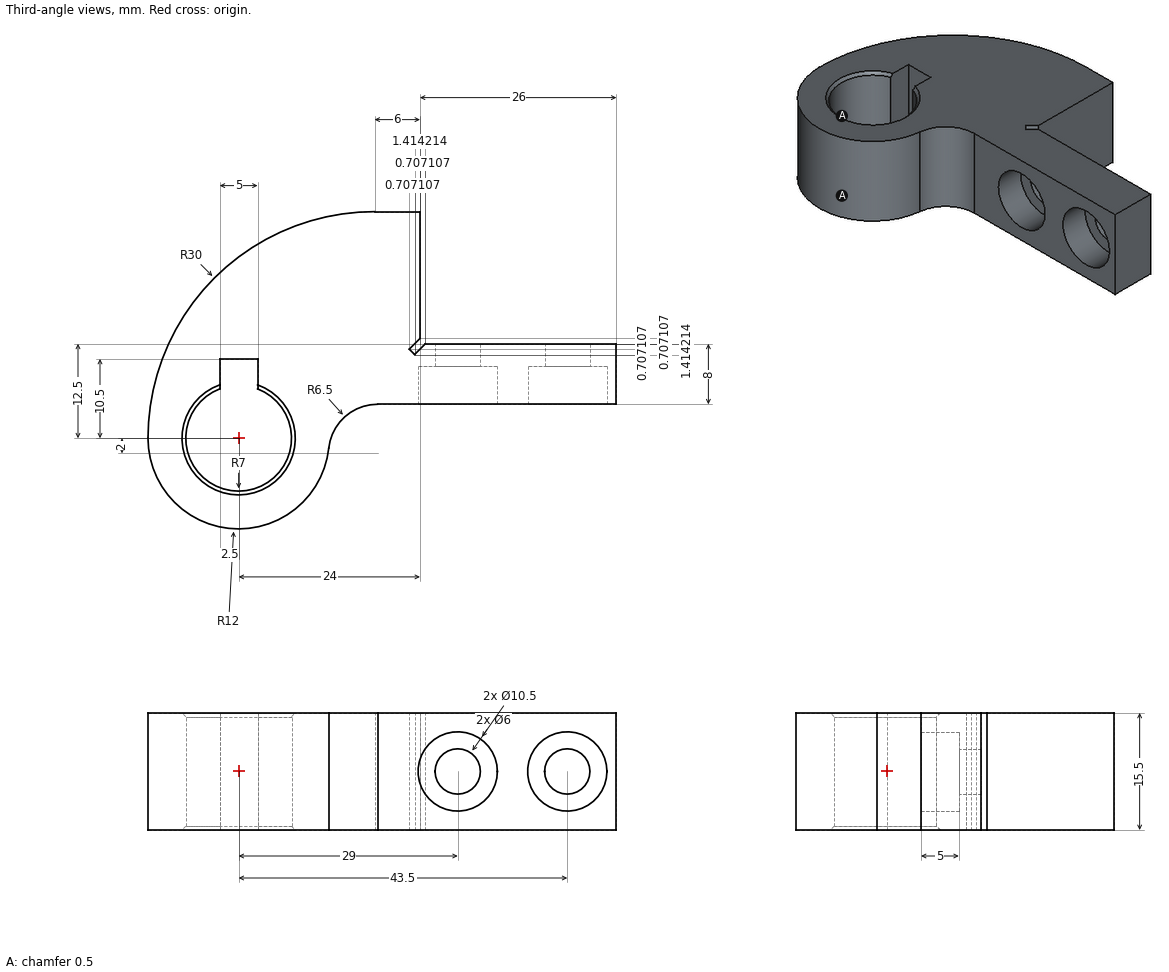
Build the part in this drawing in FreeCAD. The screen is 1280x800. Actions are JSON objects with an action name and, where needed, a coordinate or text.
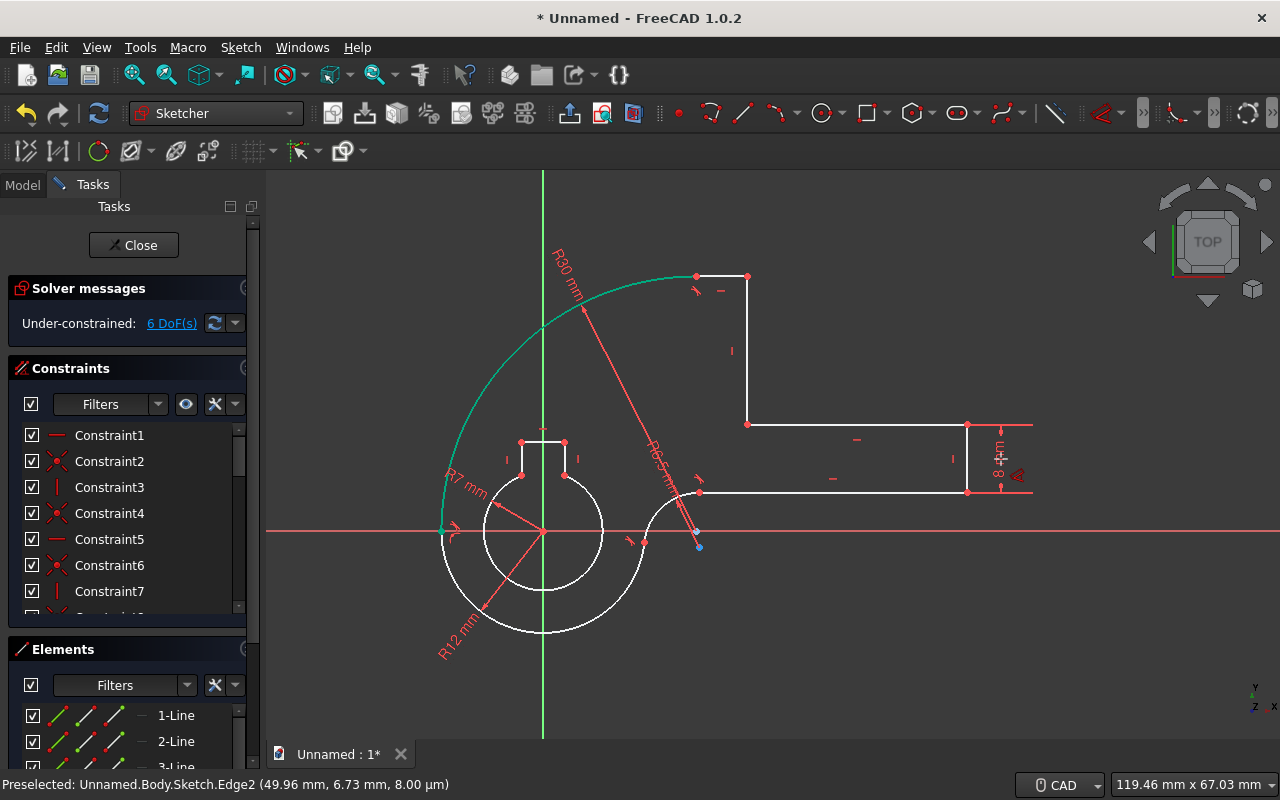
{"action": "left_click", "coordinate": [732, 276]}
{"action": "left_click", "coordinate": [722, 242]}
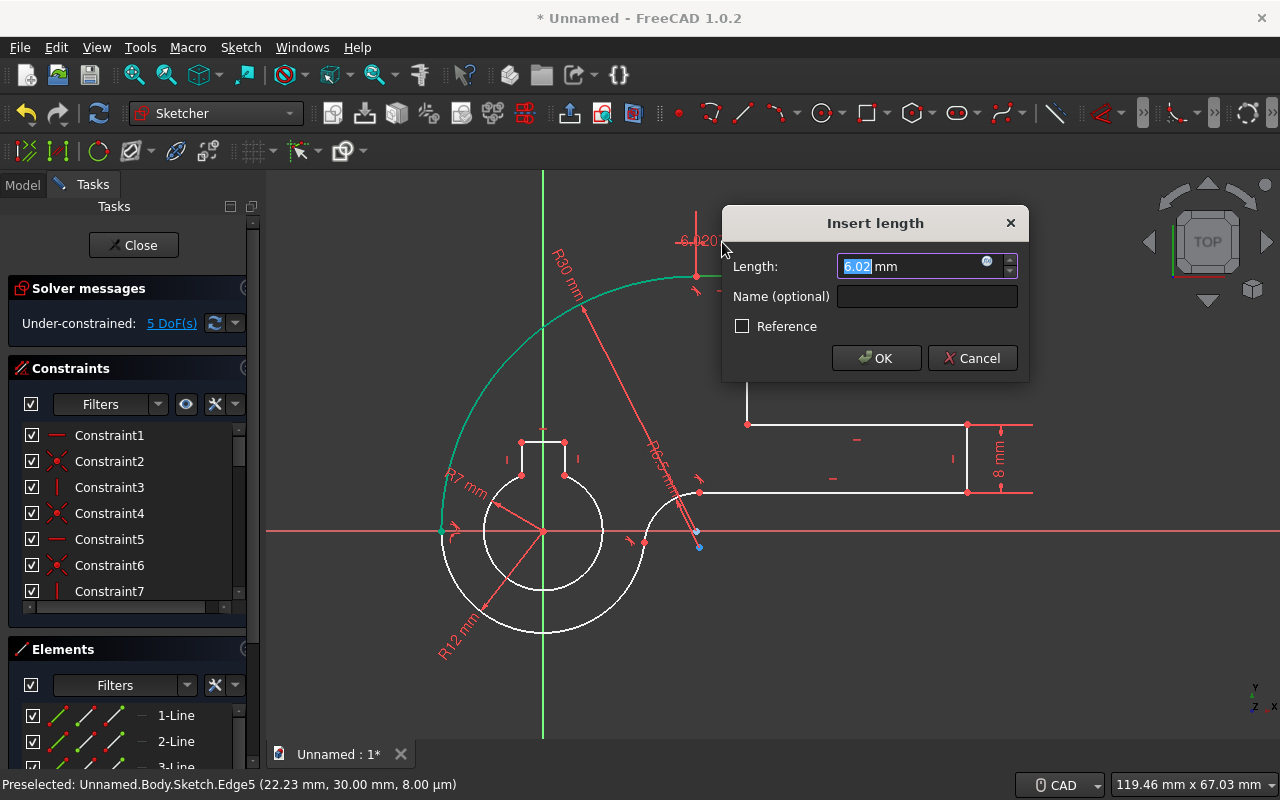
{"action": "type", "text": "6"}
{"action": "key", "text": "Return"}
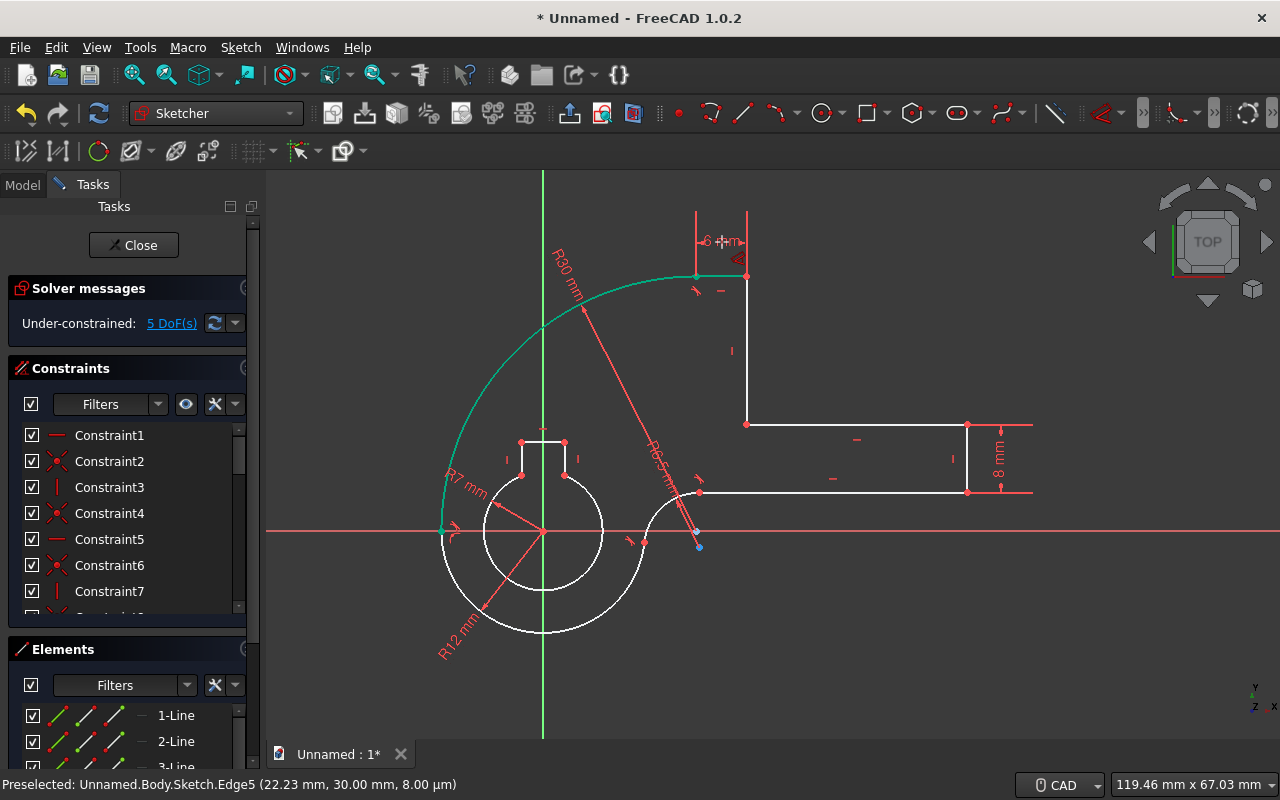
{"action": "left_click", "coordinate": [543, 442]}
{"action": "left_click", "coordinate": [528, 408]}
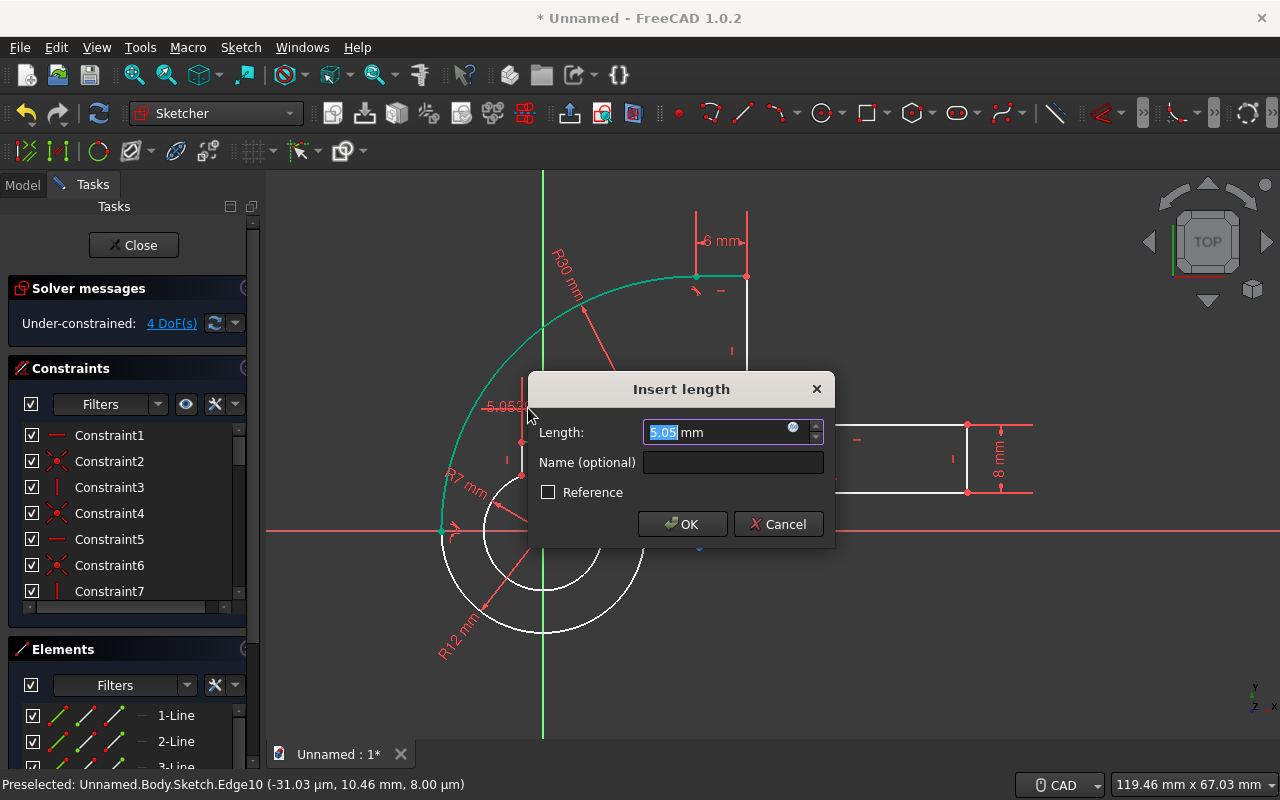
{"action": "type", "text": "5"}
{"action": "key", "text": "Return"}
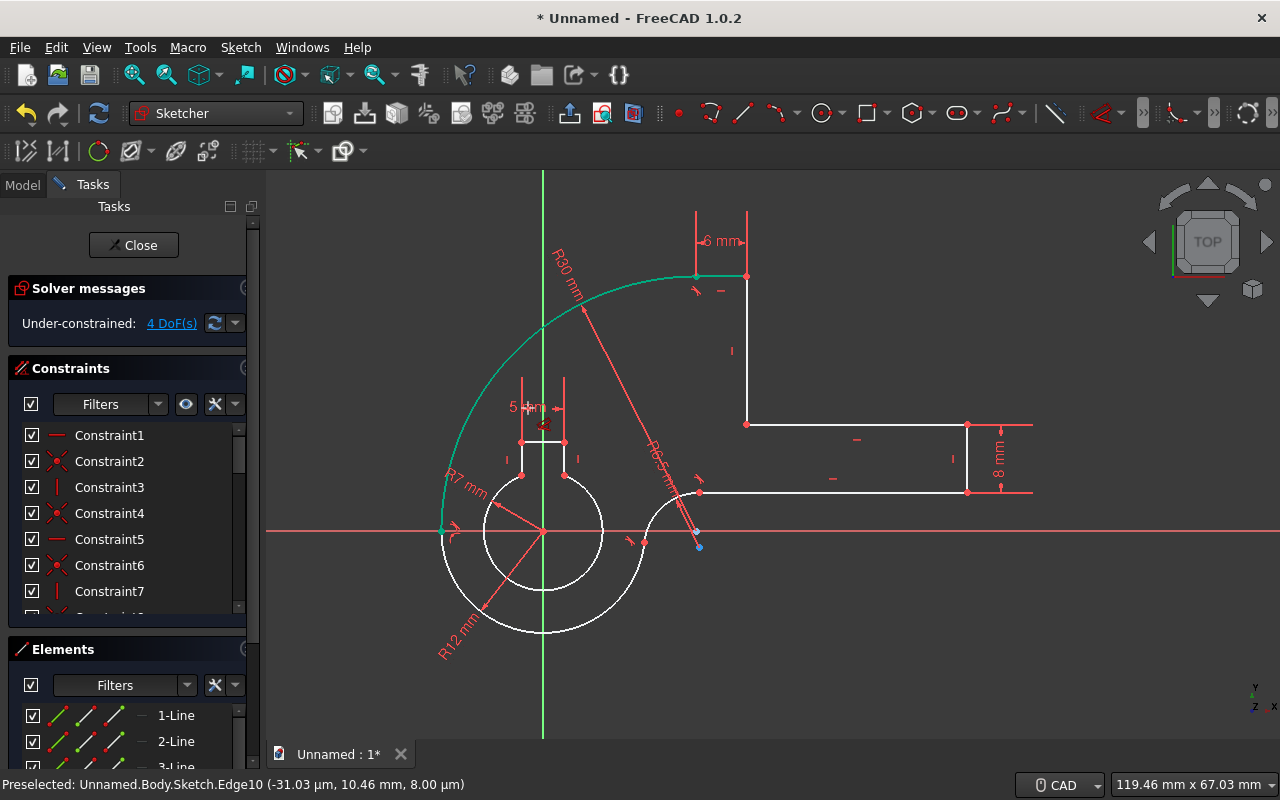
{"action": "left_click", "coordinate": [901, 425]}
{"action": "left_click", "coordinate": [857, 391]}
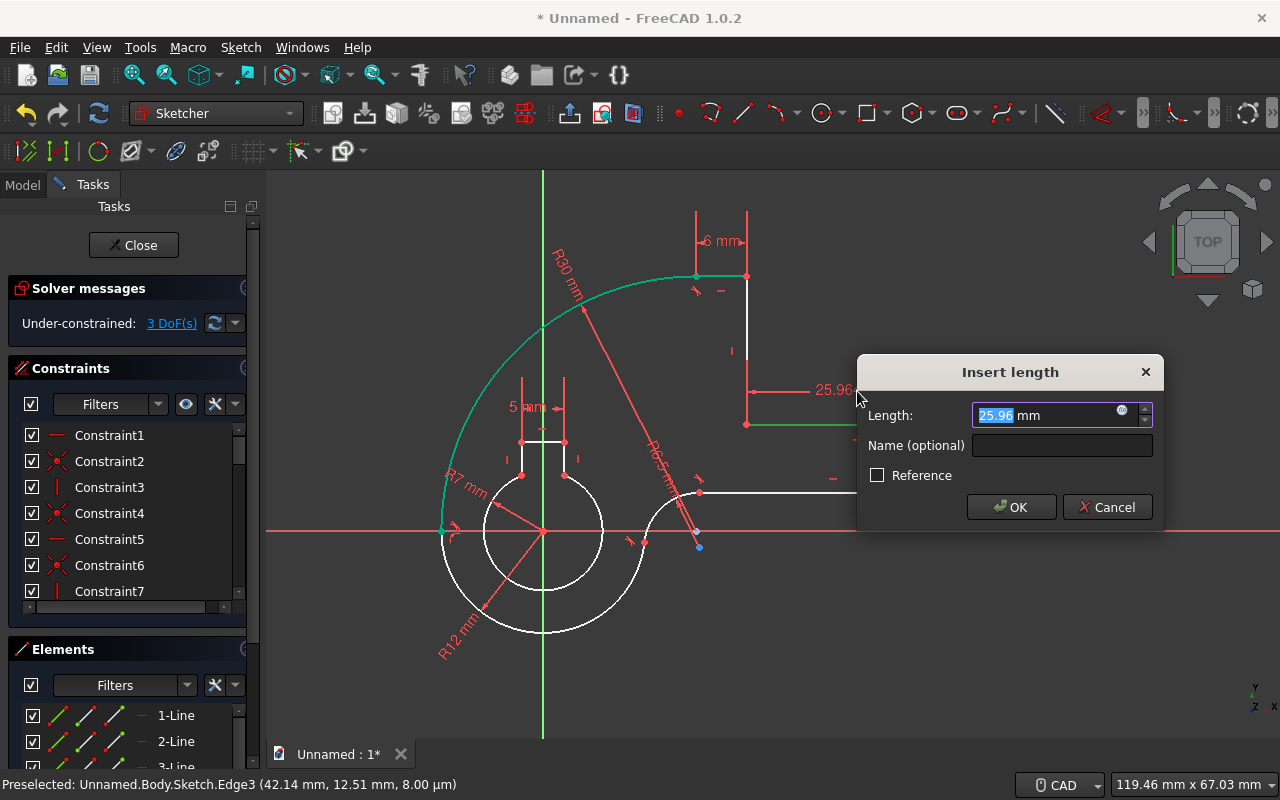
{"action": "type", "text": "26"}
{"action": "key", "text": "Return"}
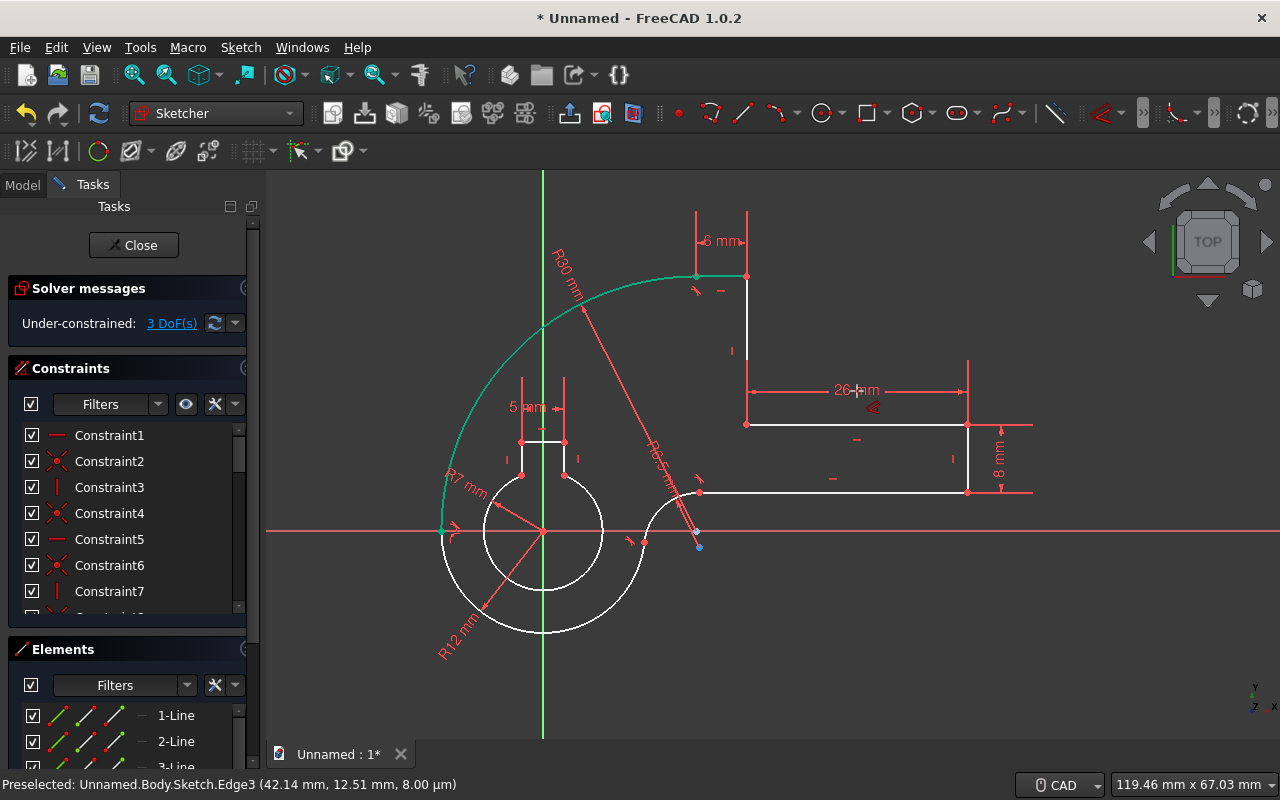
{"action": "scroll", "coordinate": [699, 548], "scroll_direction": "up", "scroll_amount": 5}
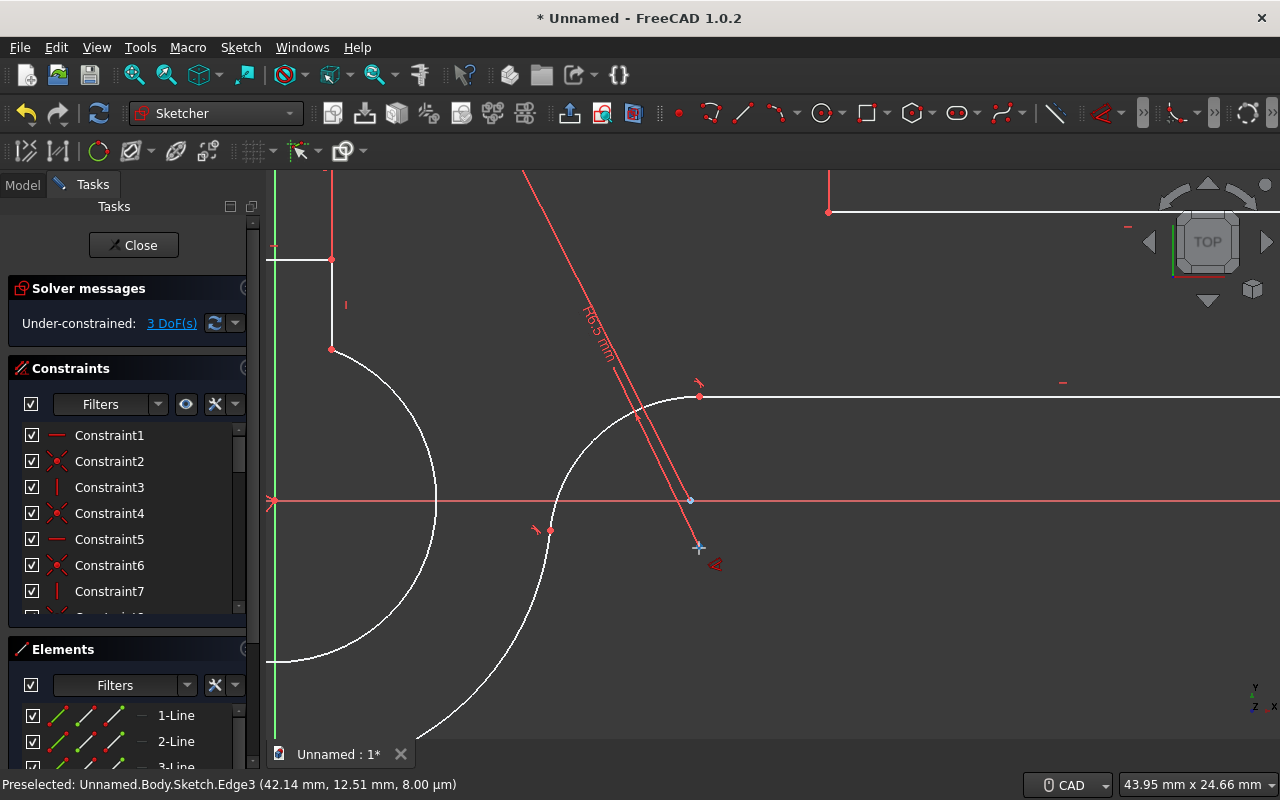
{"action": "left_click", "coordinate": [699, 547]}
{"action": "left_click", "coordinate": [733, 524]}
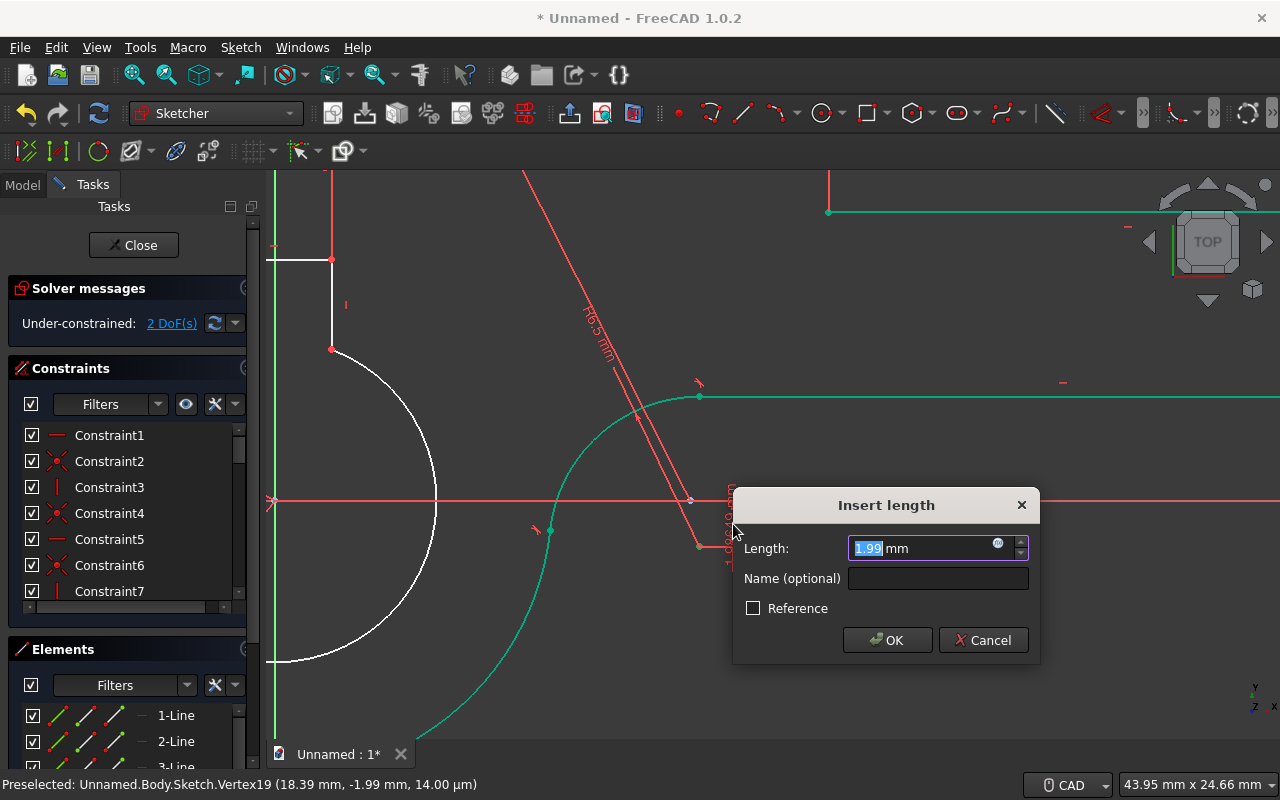
{"action": "type", "text": "2"}
{"action": "key", "text": "Return"}